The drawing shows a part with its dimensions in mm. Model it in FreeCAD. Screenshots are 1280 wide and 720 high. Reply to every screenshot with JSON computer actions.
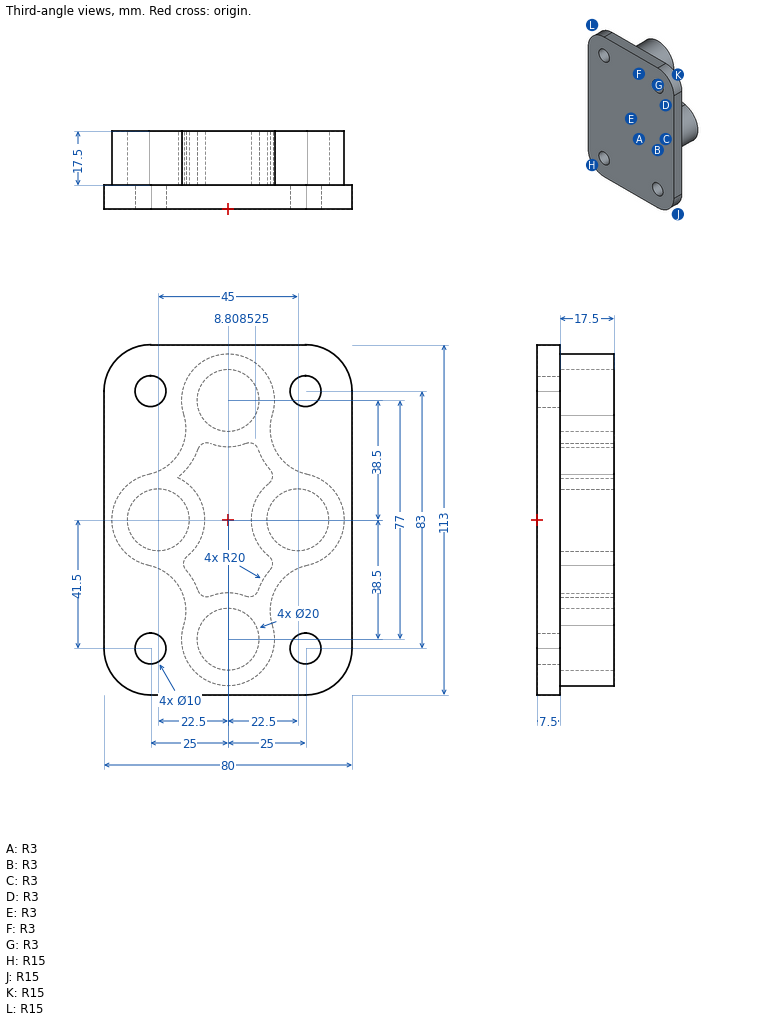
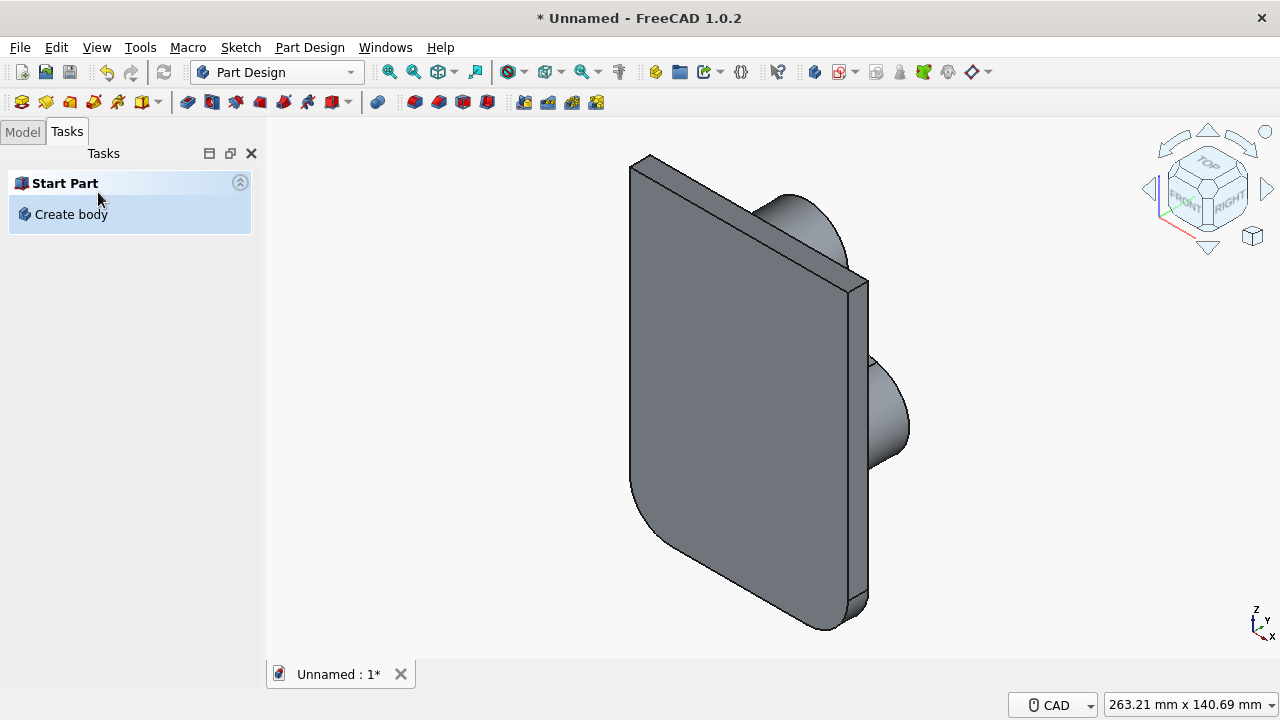
{"action": "left_click", "coordinate": [858, 286]}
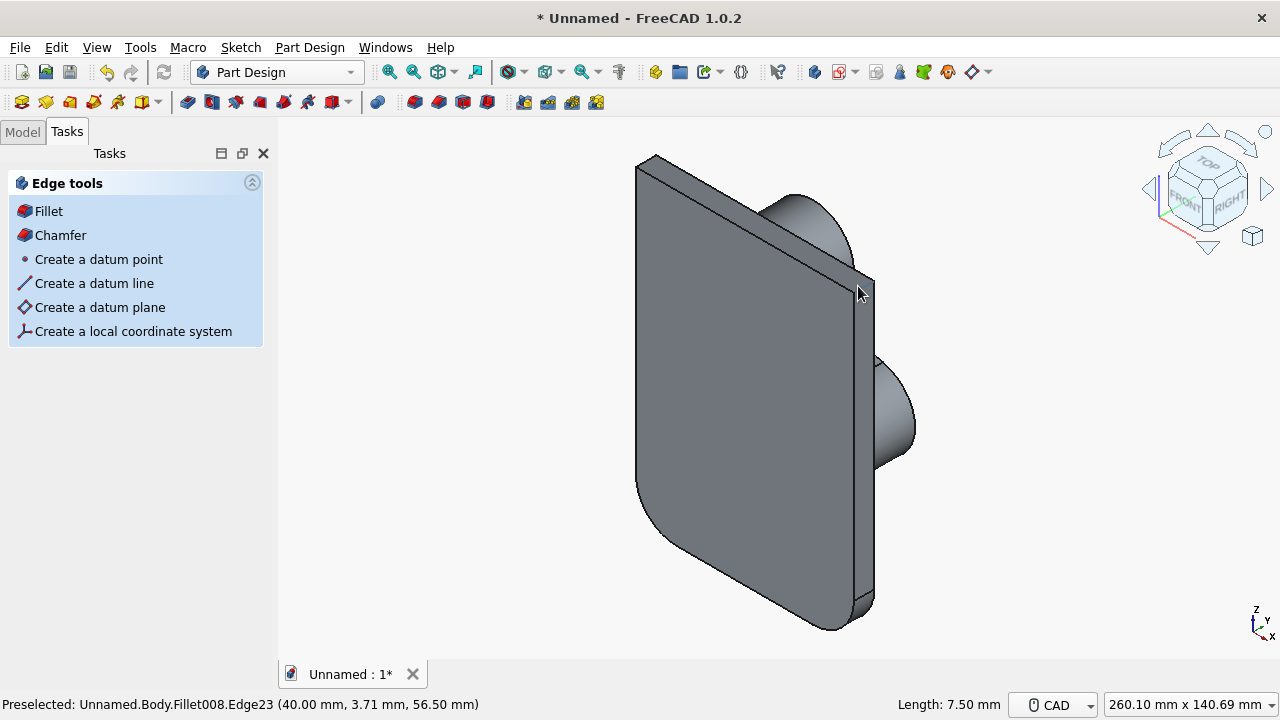
{"action": "left_click", "coordinate": [416, 102]}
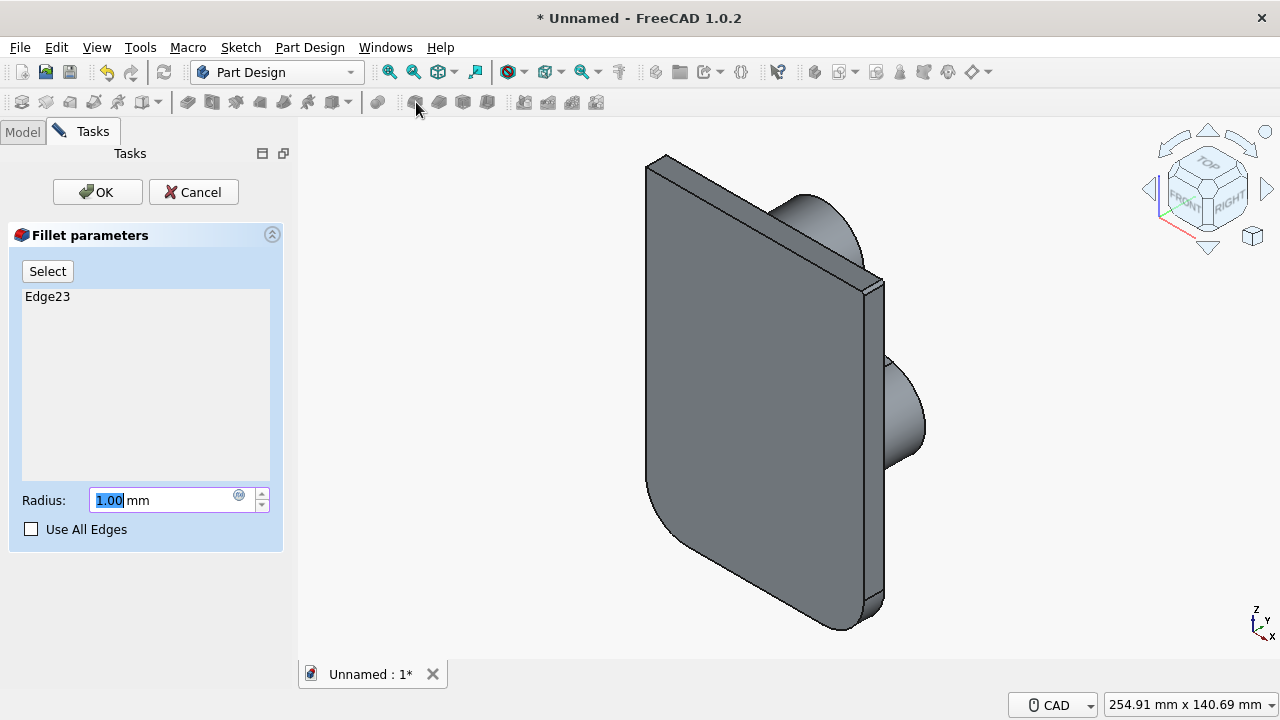
{"action": "type", "text": "15"}
{"action": "key", "text": "Tab"}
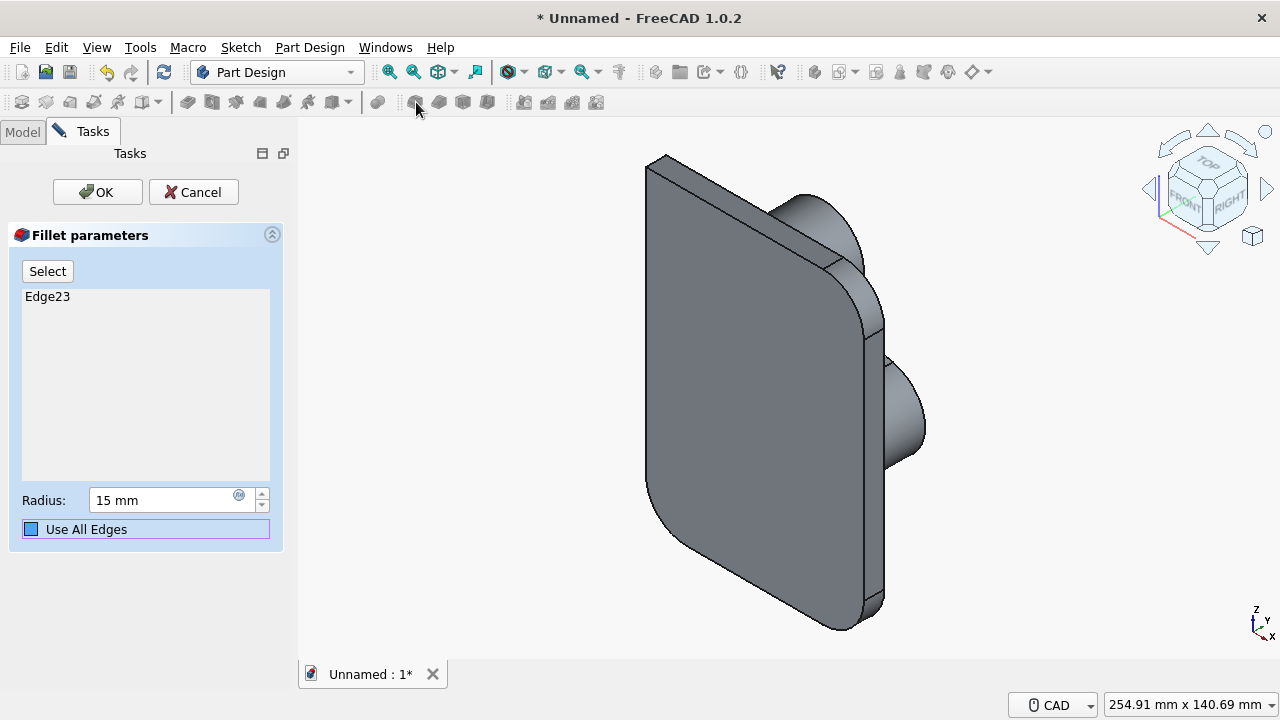
{"action": "left_click", "coordinate": [98, 192]}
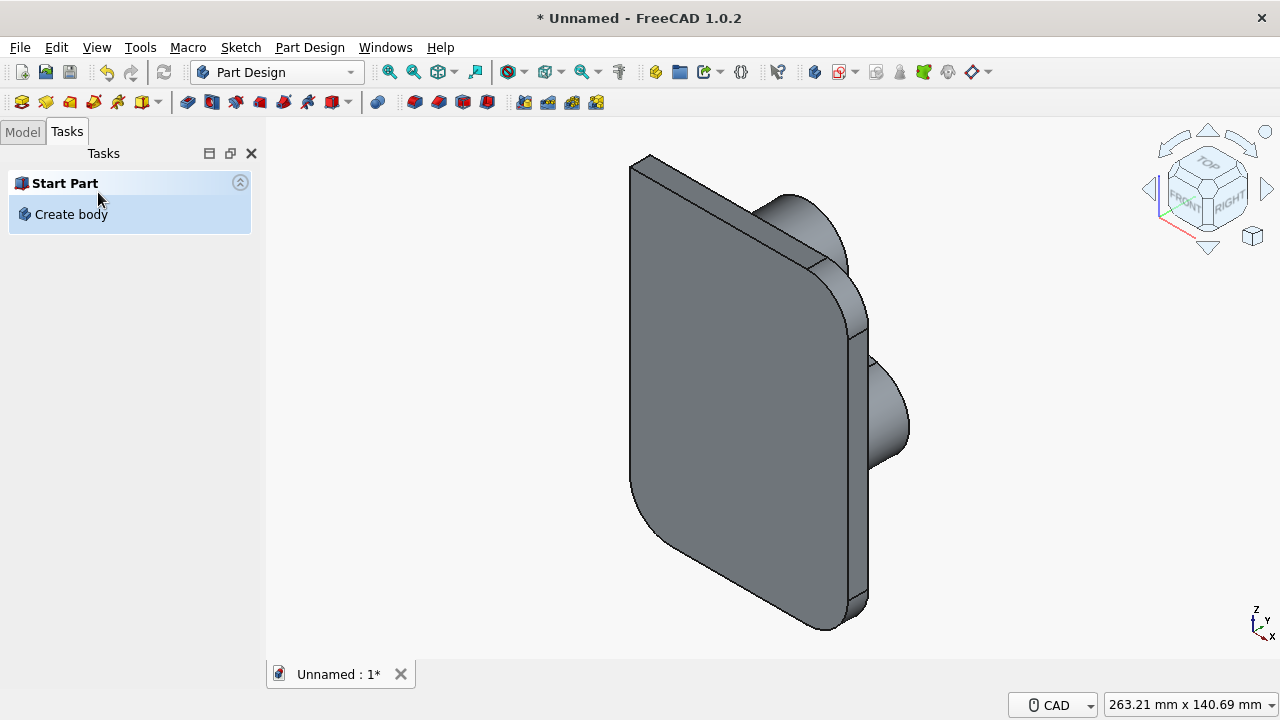
{"action": "key", "text": "2"}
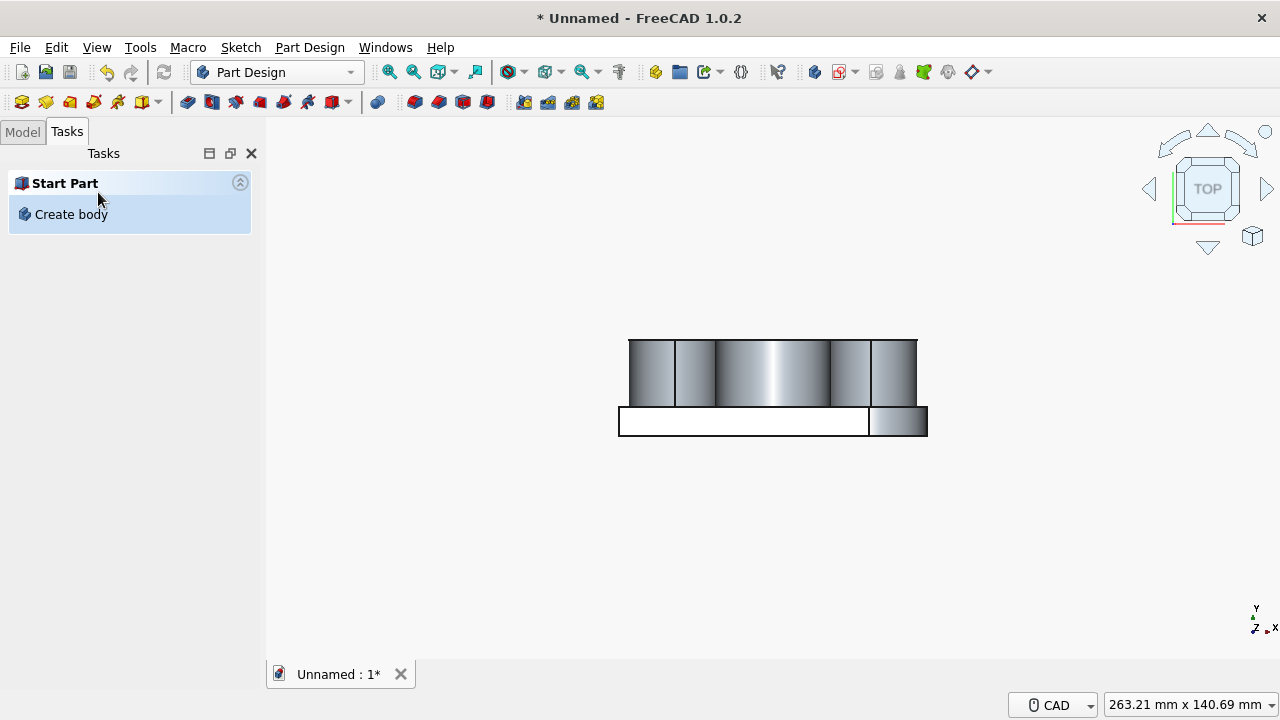
{"action": "key", "text": "v f"}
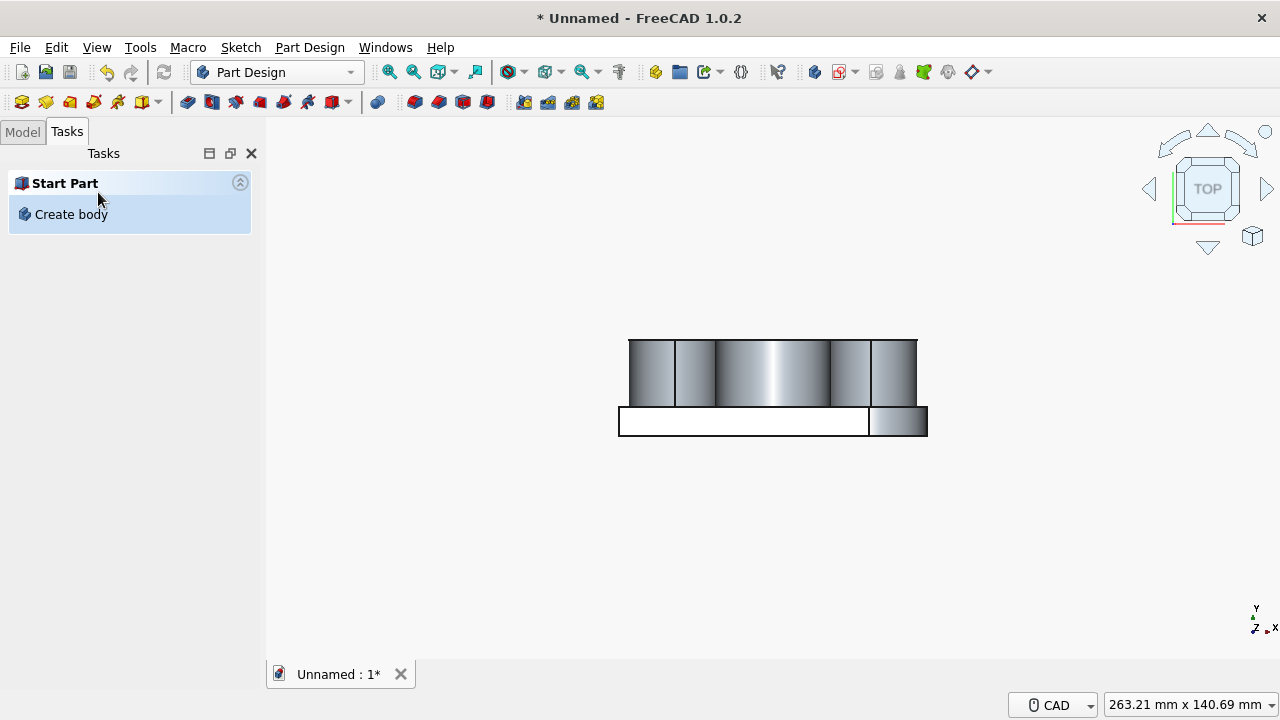
{"action": "left_click", "coordinate": [619, 421]}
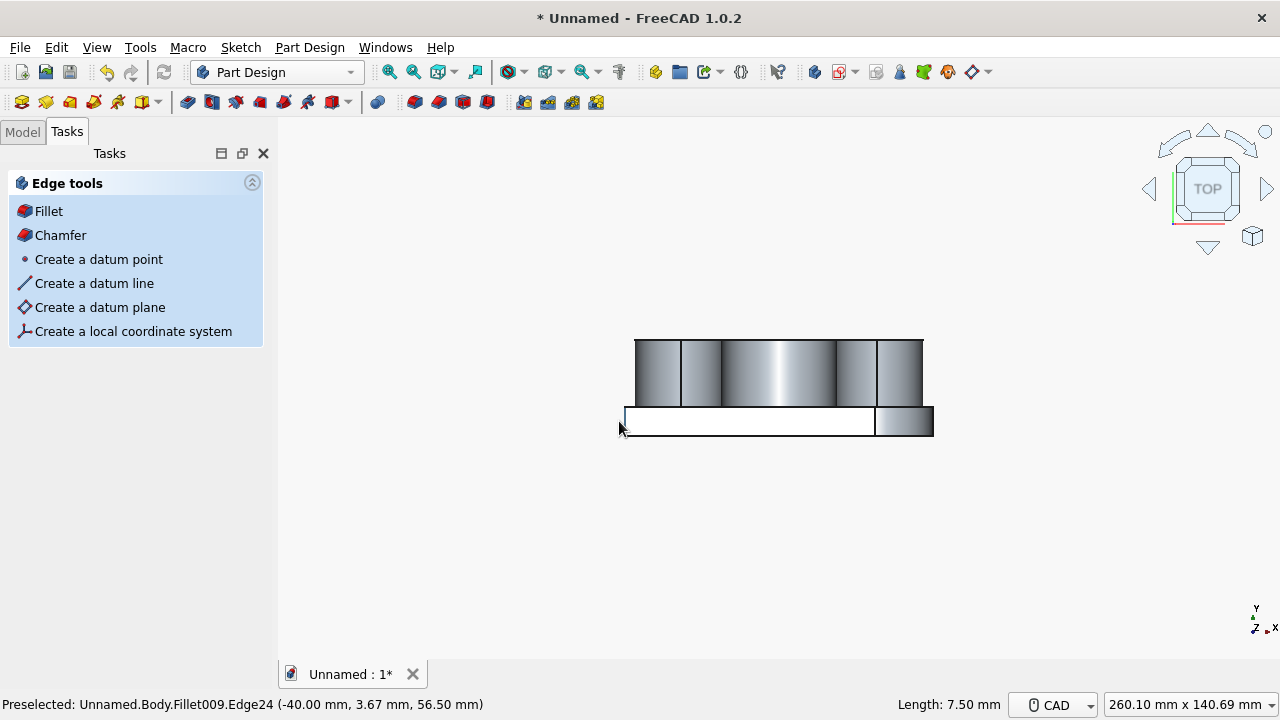
{"action": "left_click", "coordinate": [416, 102]}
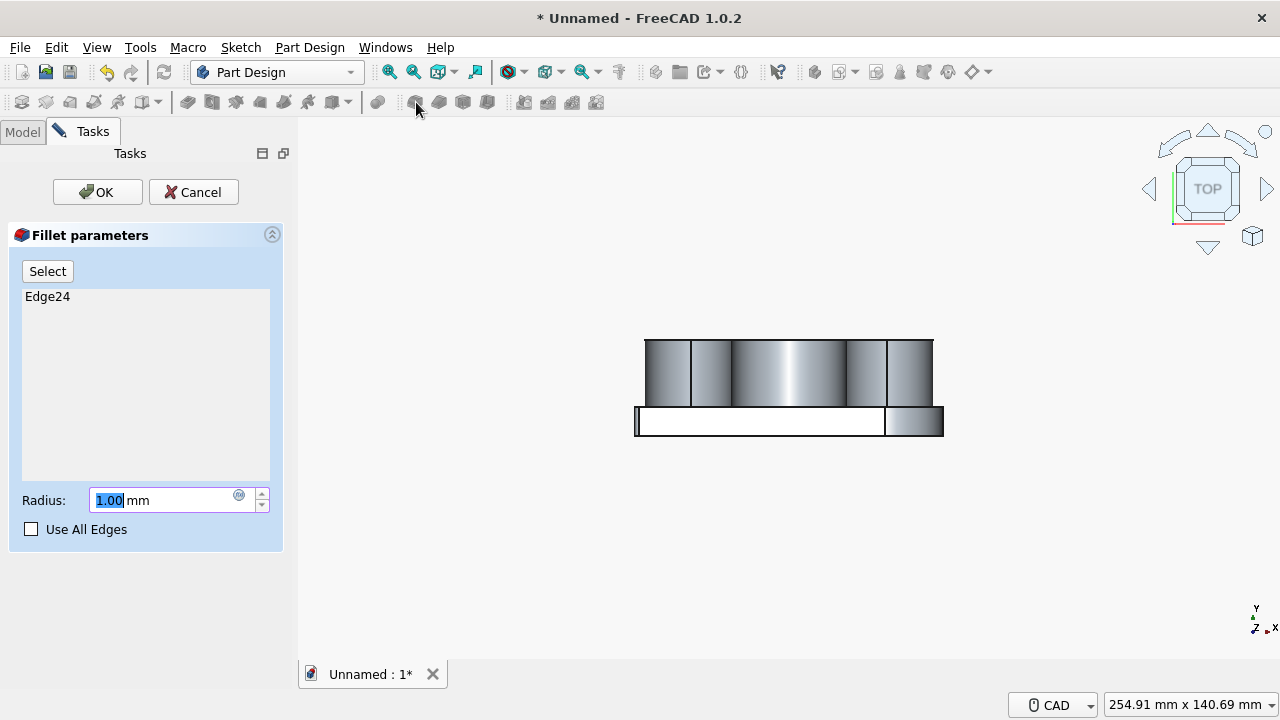
{"action": "type", "text": "15"}
{"action": "key", "text": "Tab"}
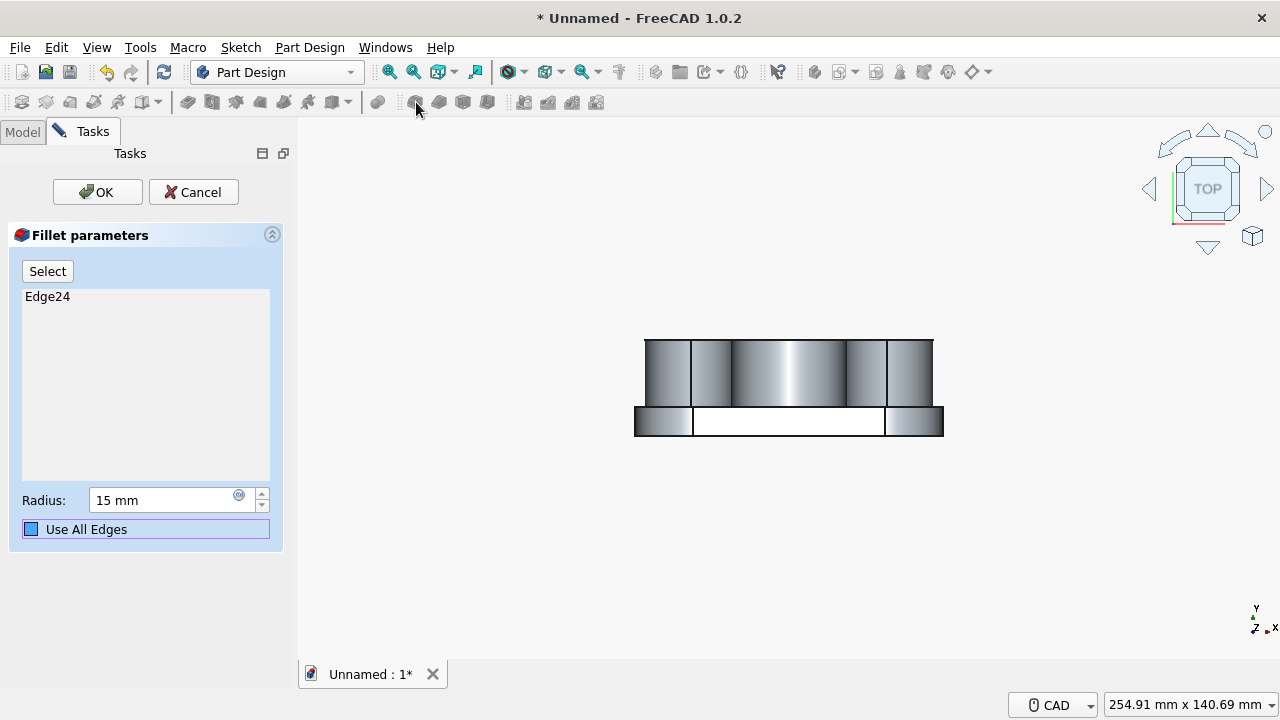
{"action": "left_click", "coordinate": [98, 192]}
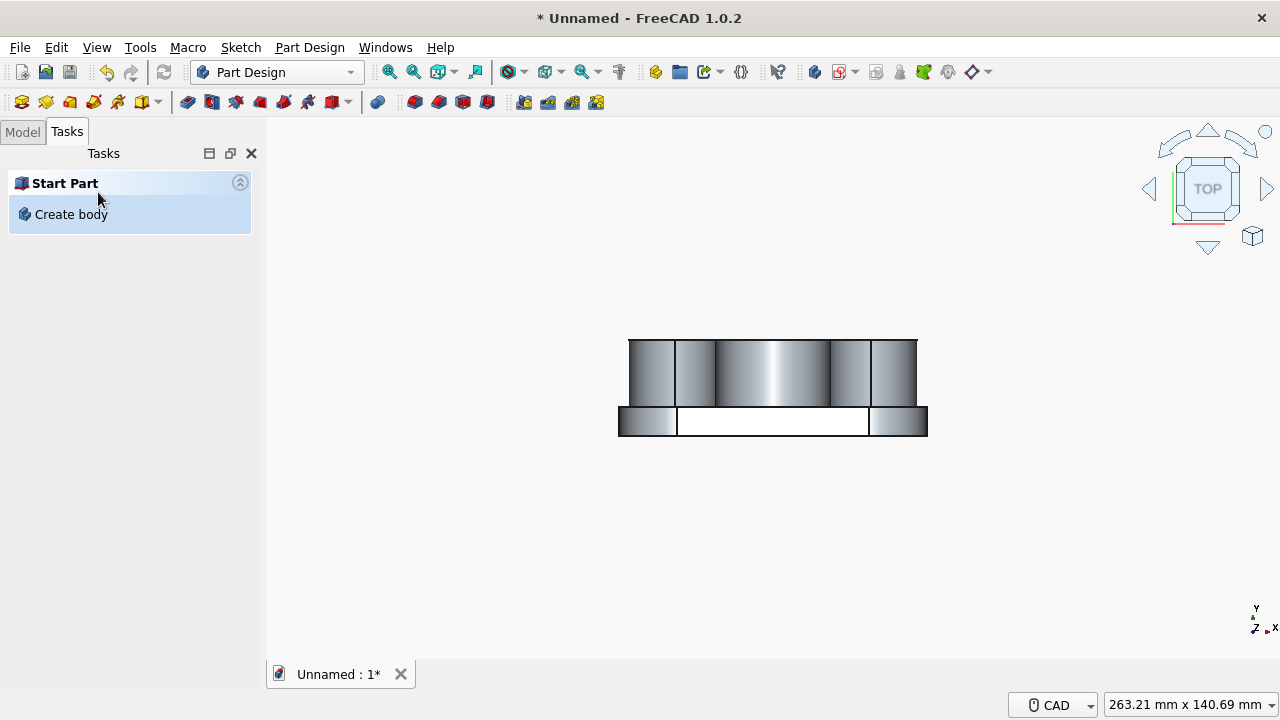
{"action": "left_click", "coordinate": [390, 72]}